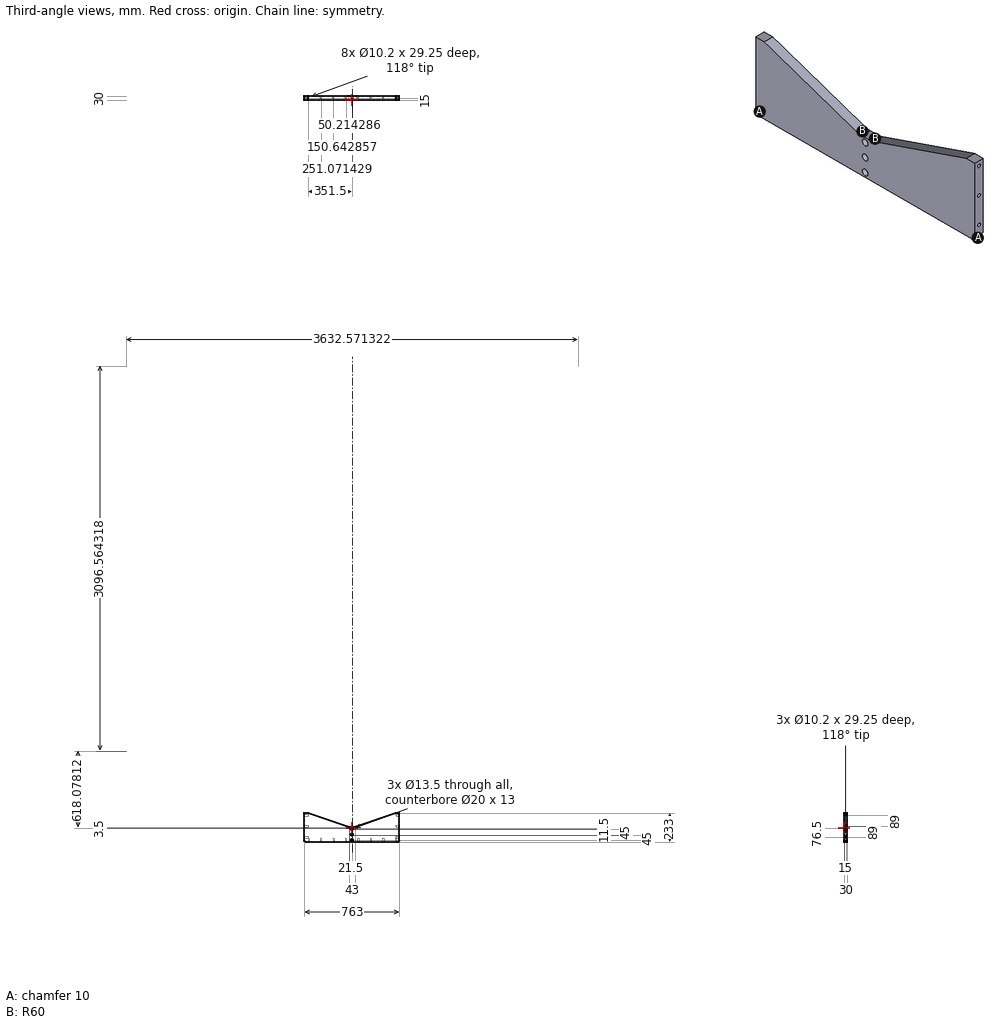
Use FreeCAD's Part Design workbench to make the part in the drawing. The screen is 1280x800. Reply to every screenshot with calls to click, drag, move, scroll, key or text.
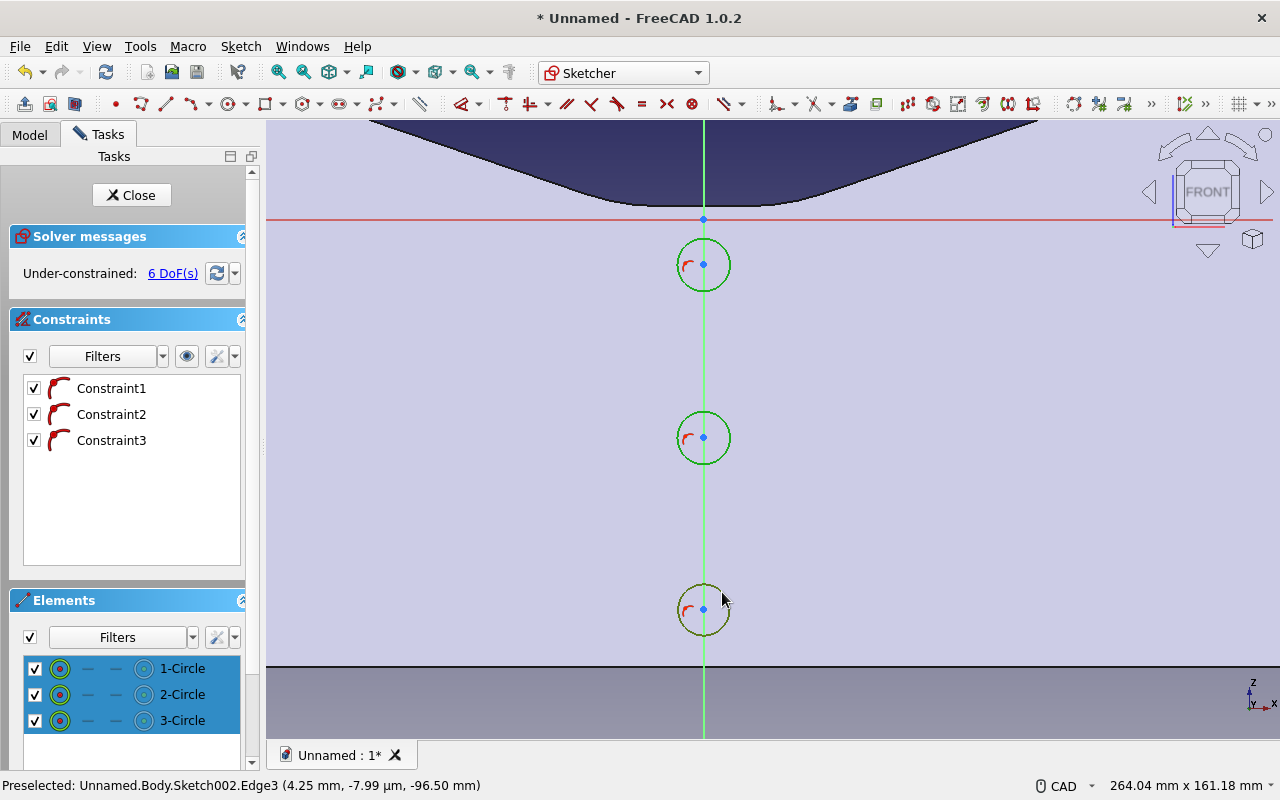
key(e)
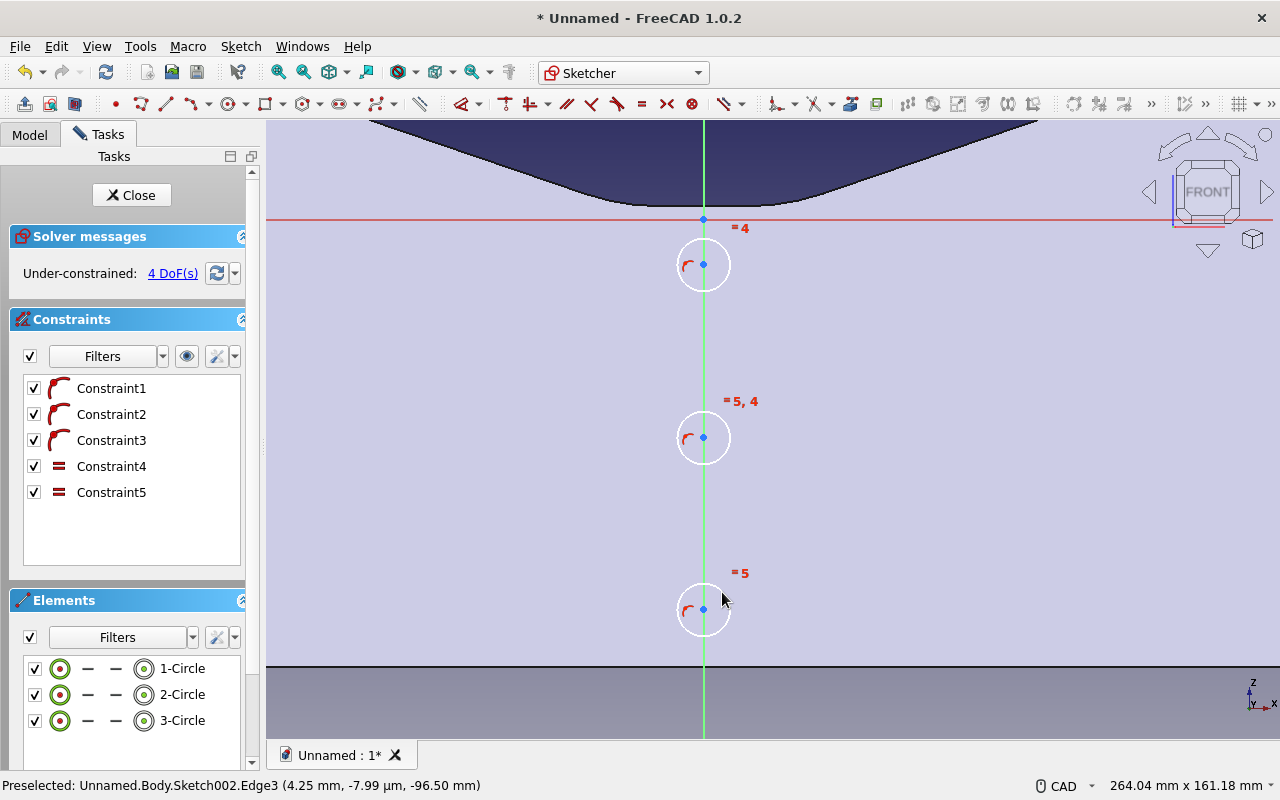
key(d)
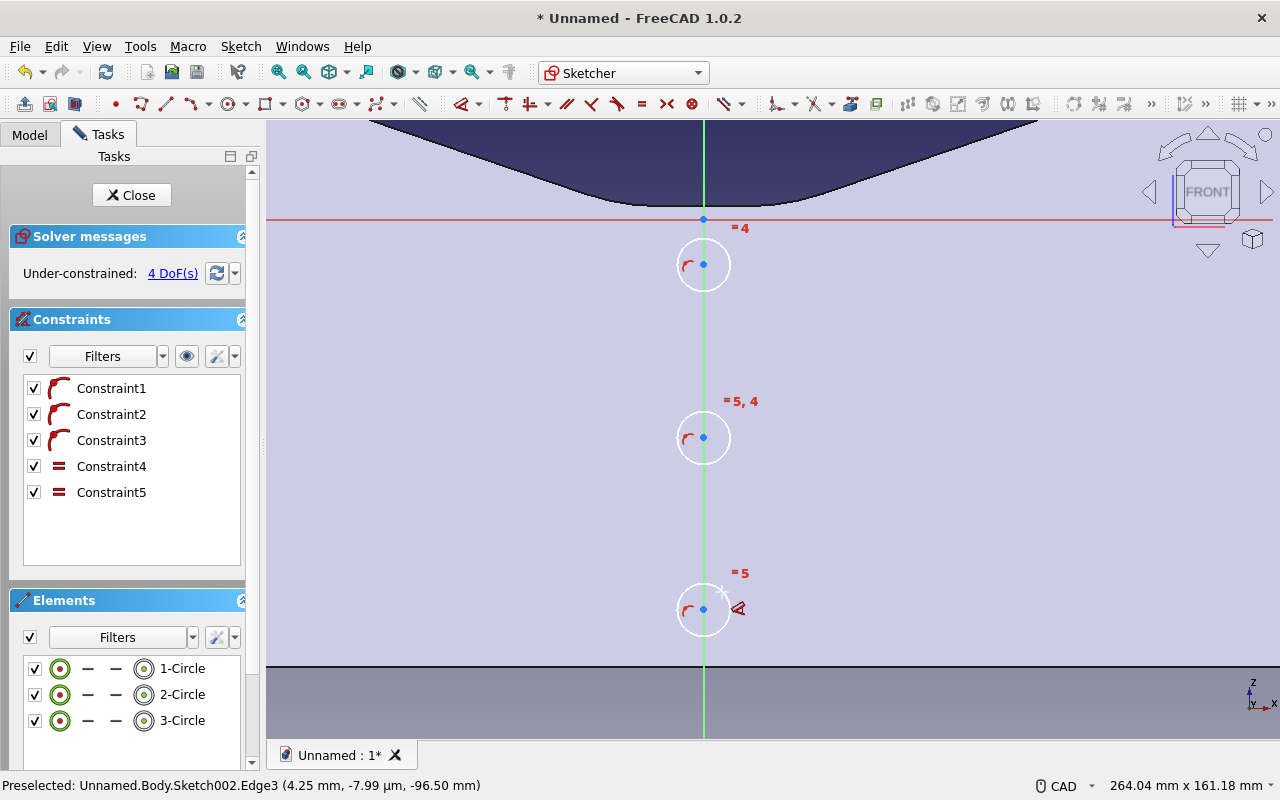
click(722, 246)
click(759, 247)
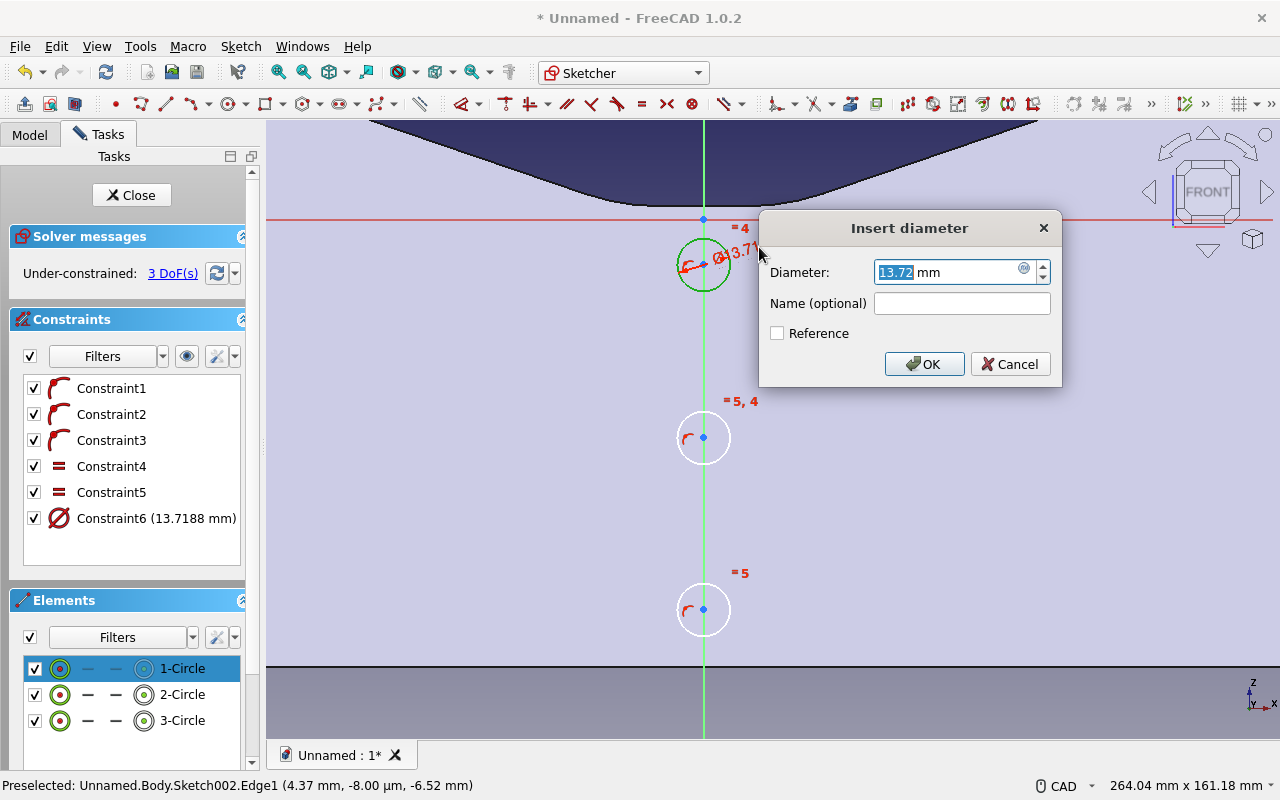
text(13.5)
key(Return)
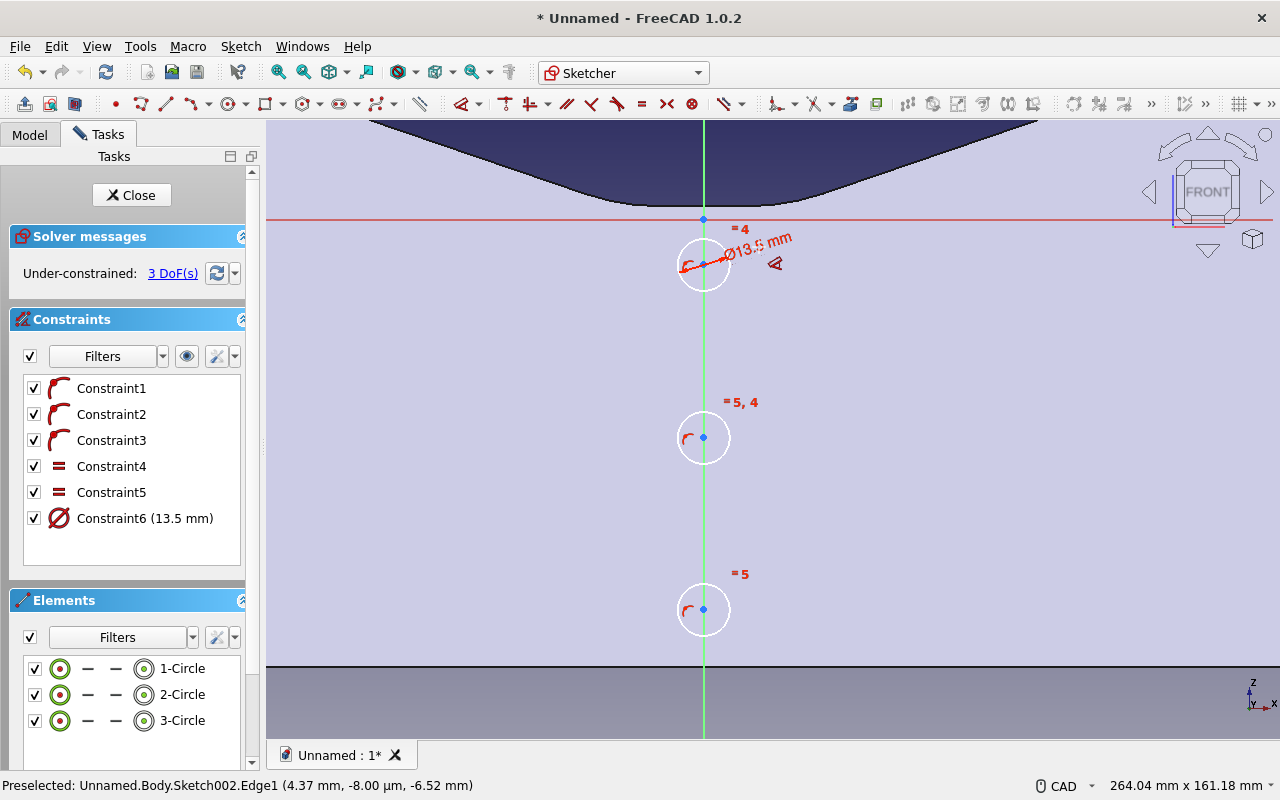
click(704, 265)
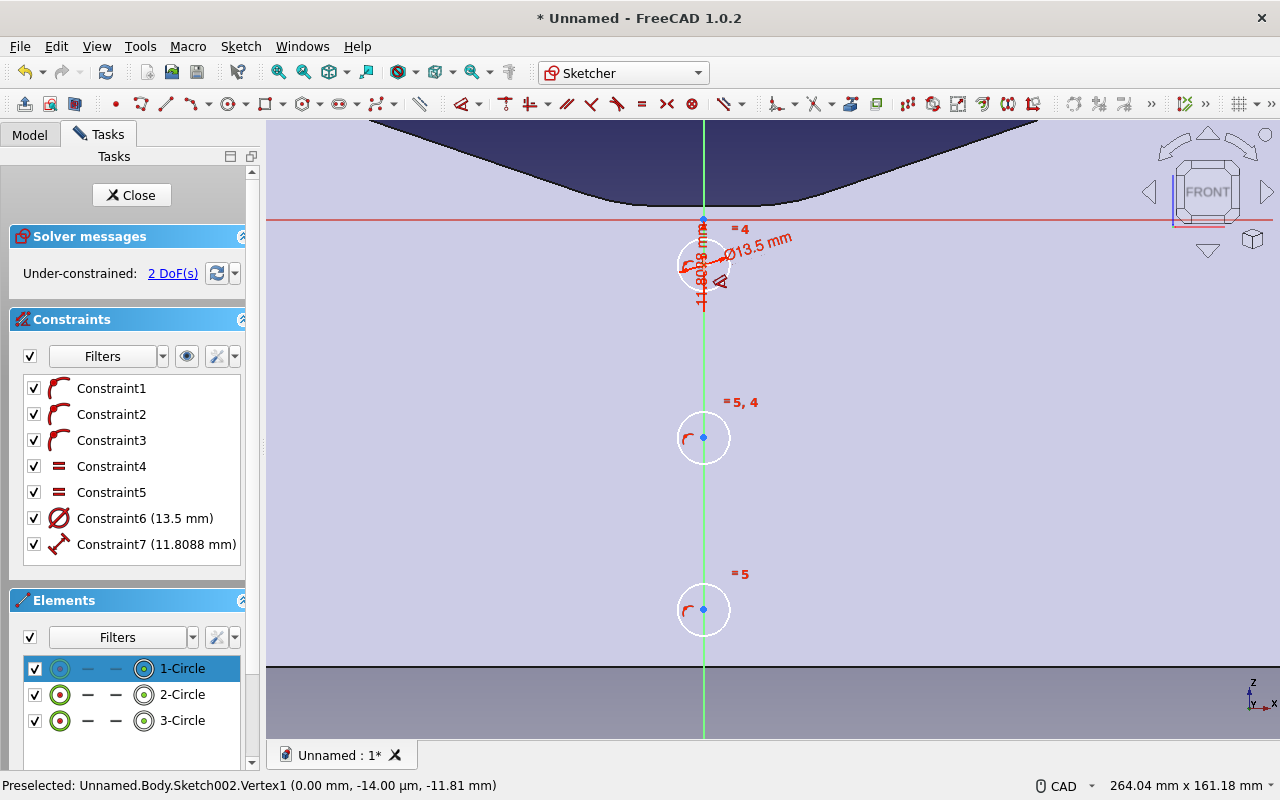
click(704, 438)
click(738, 352)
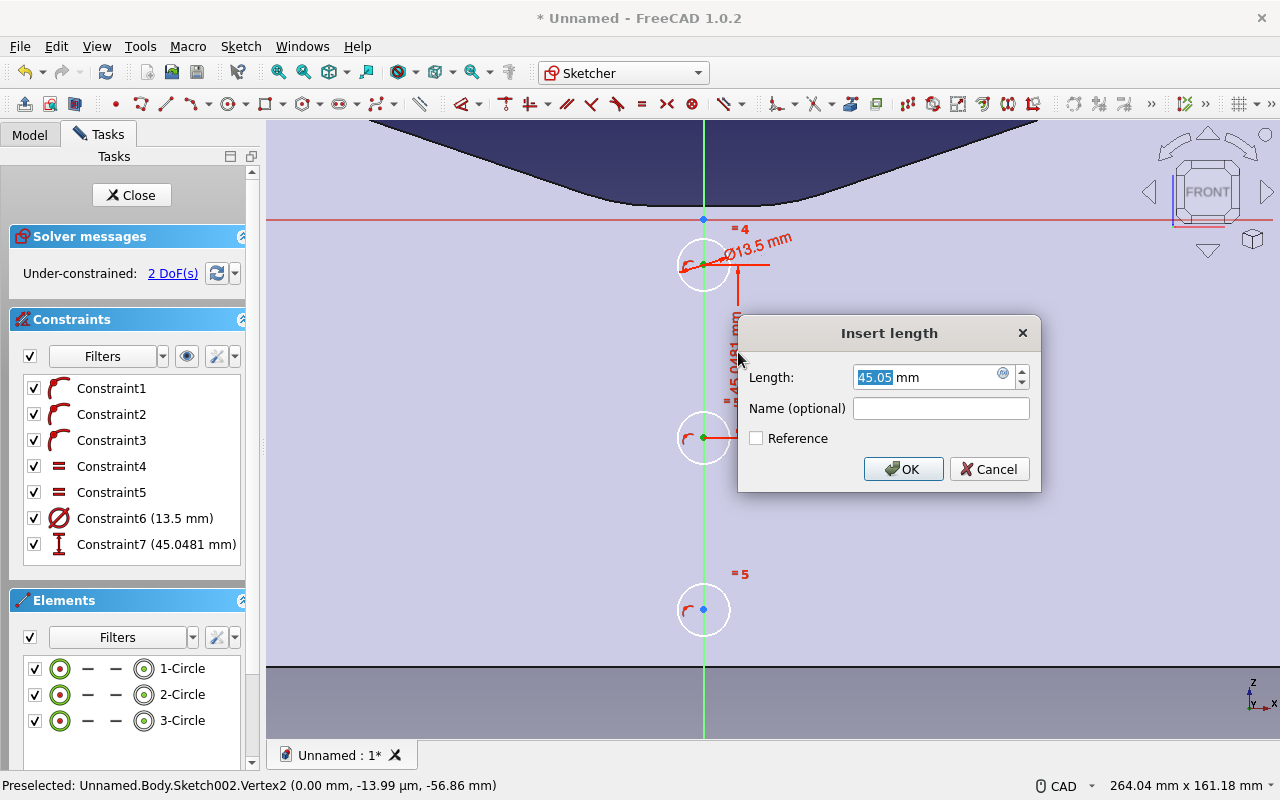
text(45)
key(Return)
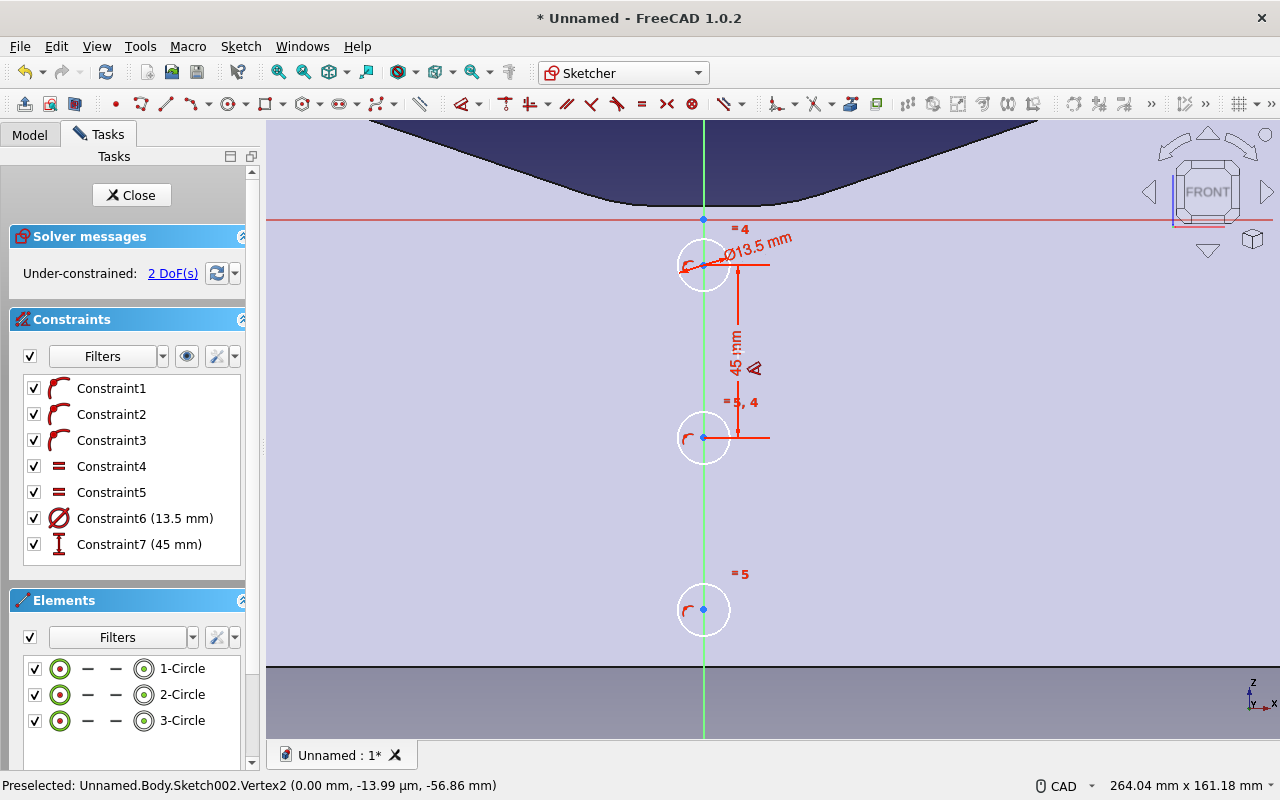
click(704, 438)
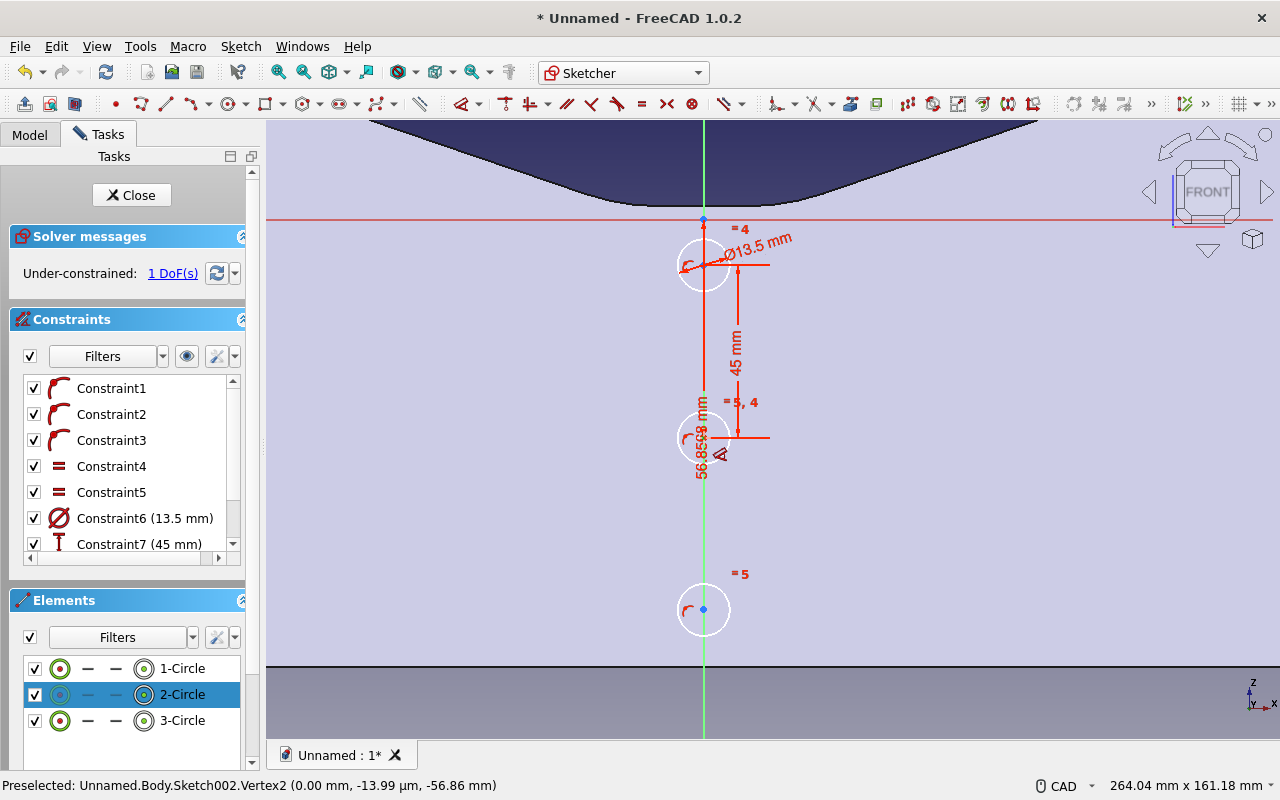
click(704, 610)
click(738, 524)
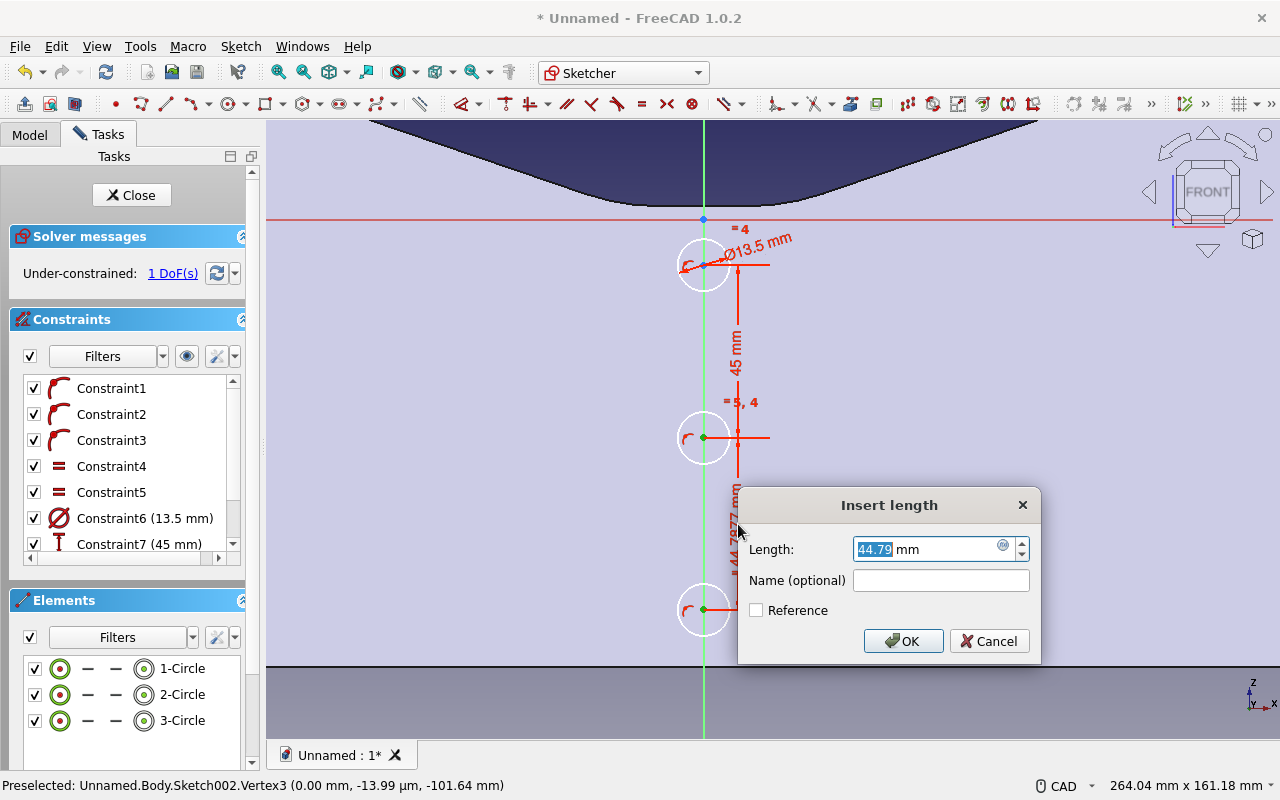
text(45)
key(Return)